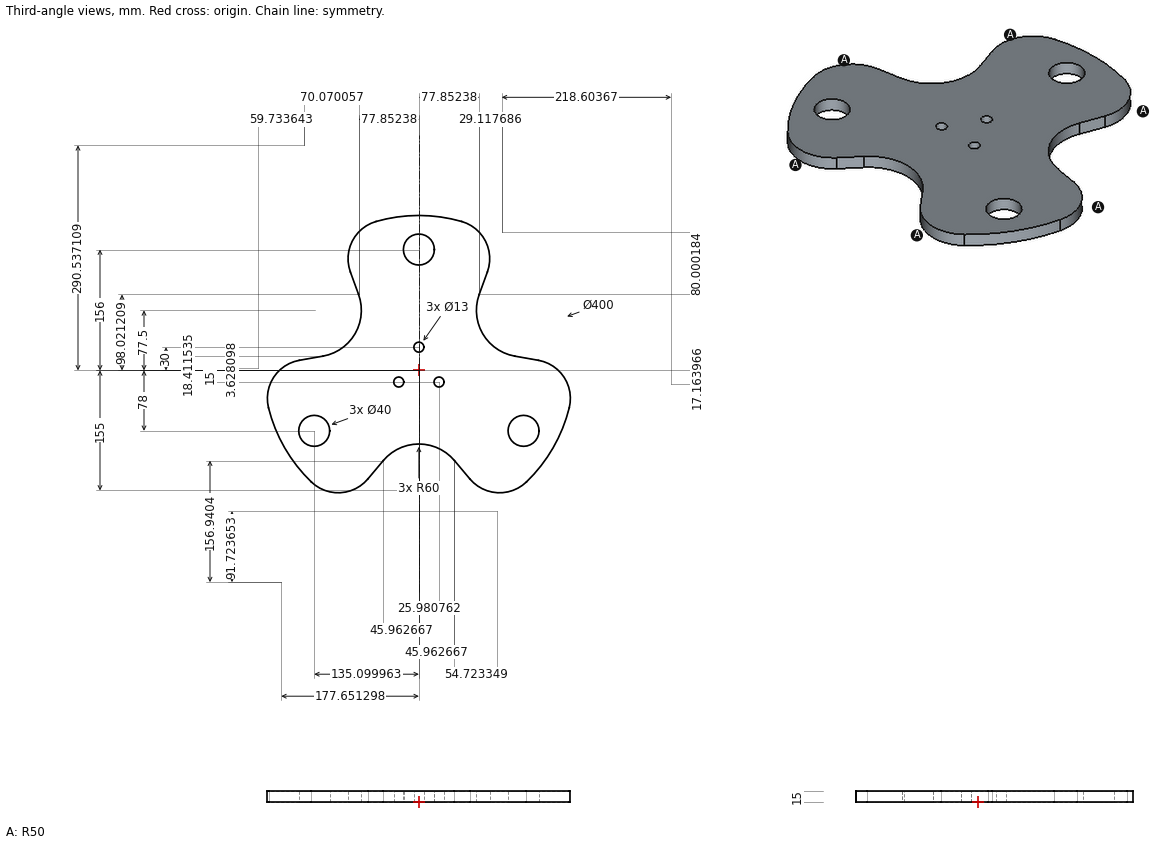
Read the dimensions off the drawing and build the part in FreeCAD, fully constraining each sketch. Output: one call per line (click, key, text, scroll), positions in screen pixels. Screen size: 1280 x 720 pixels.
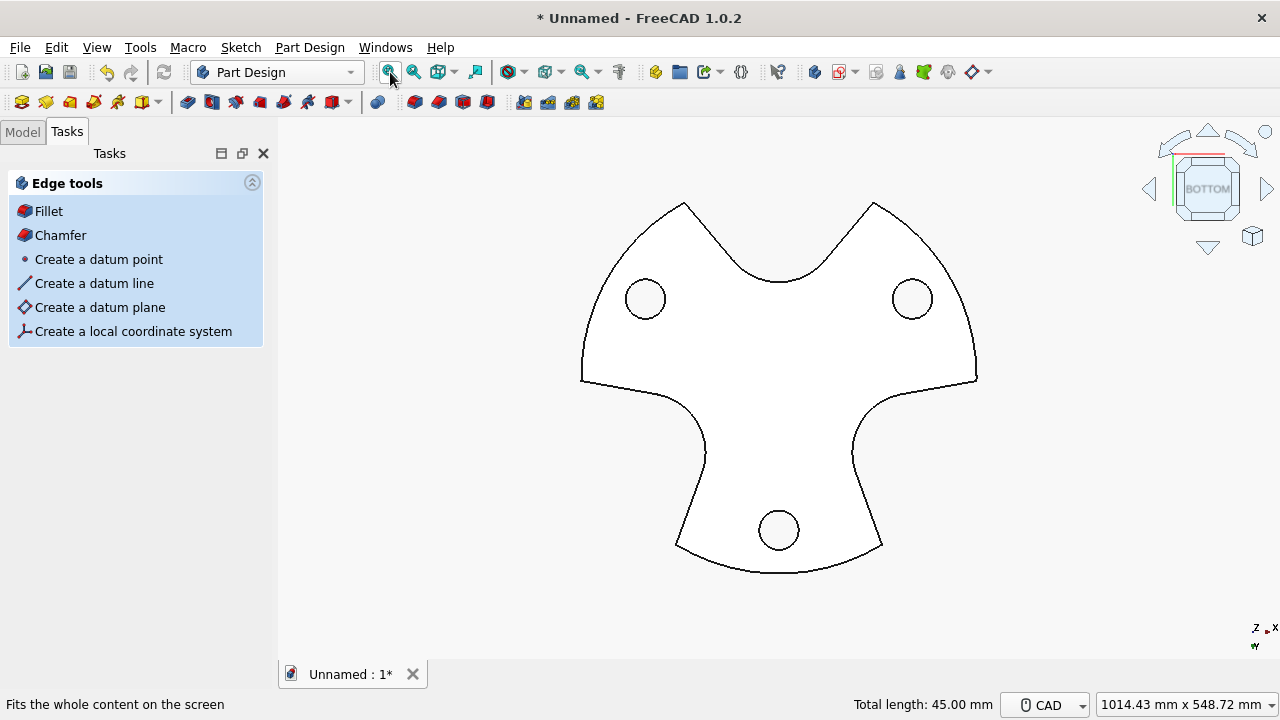
key(4)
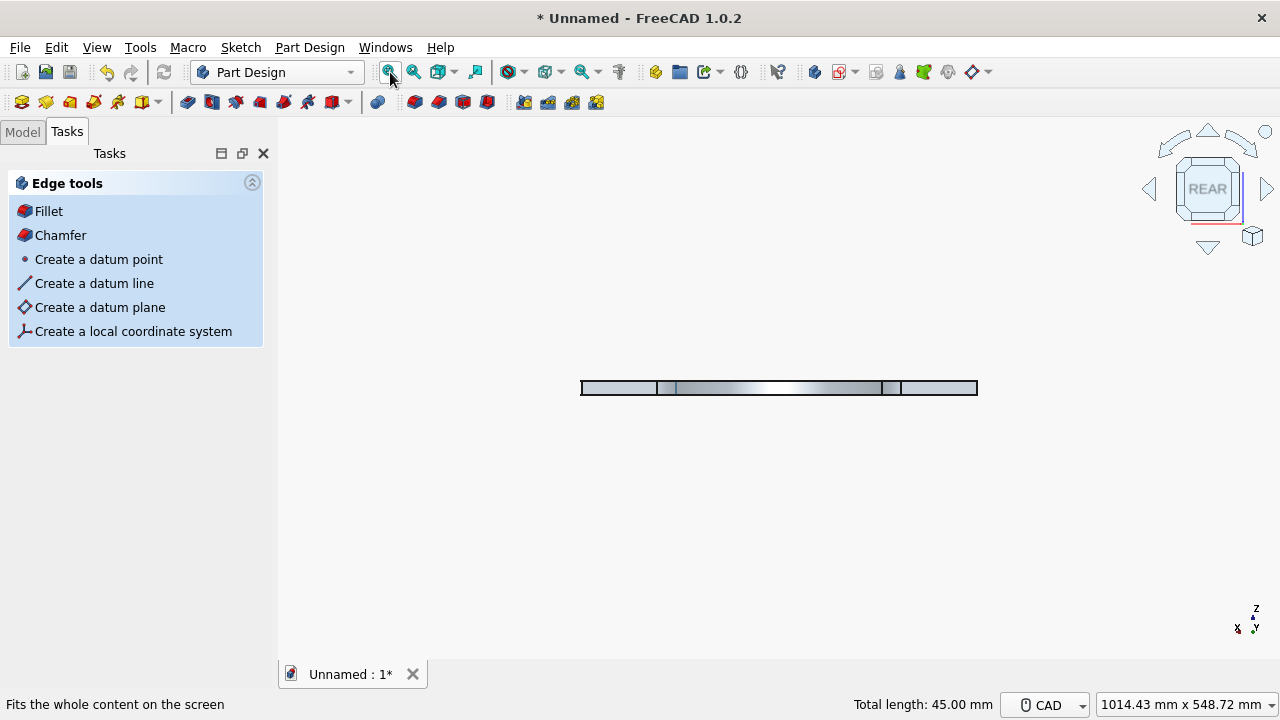
click(390, 72)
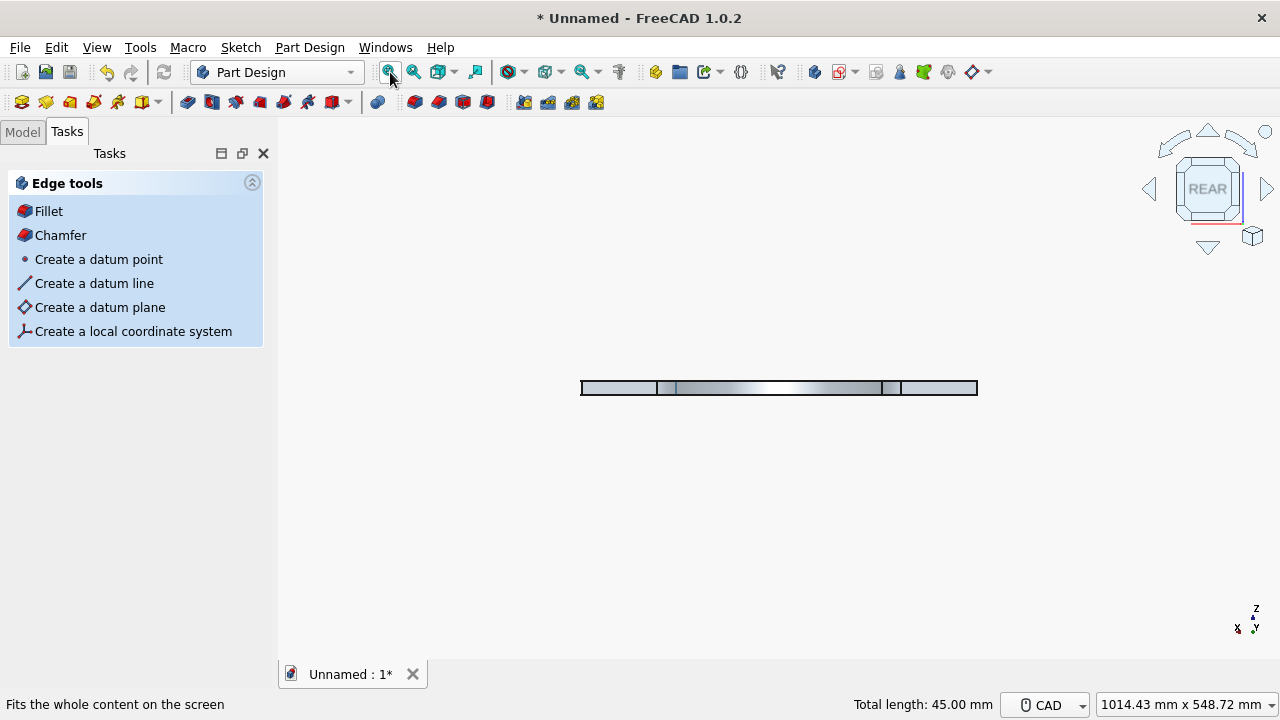
scroll(582, 387, up, 5)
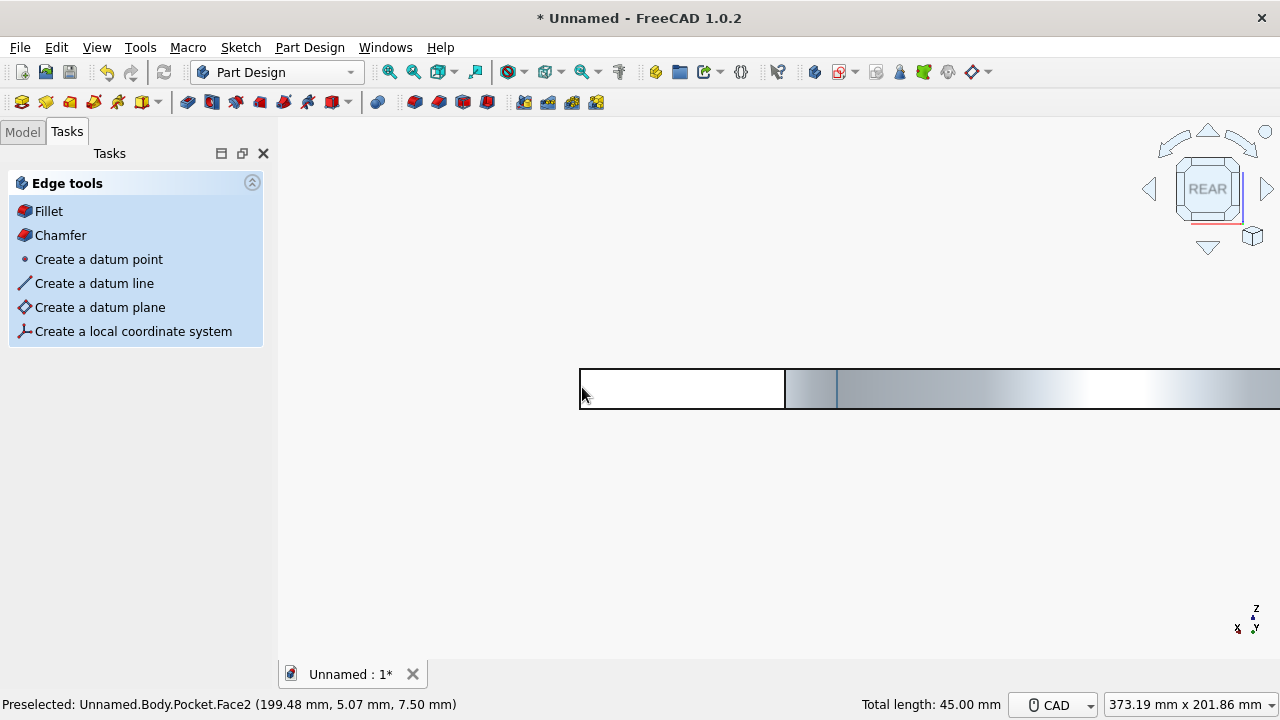
click(390, 72)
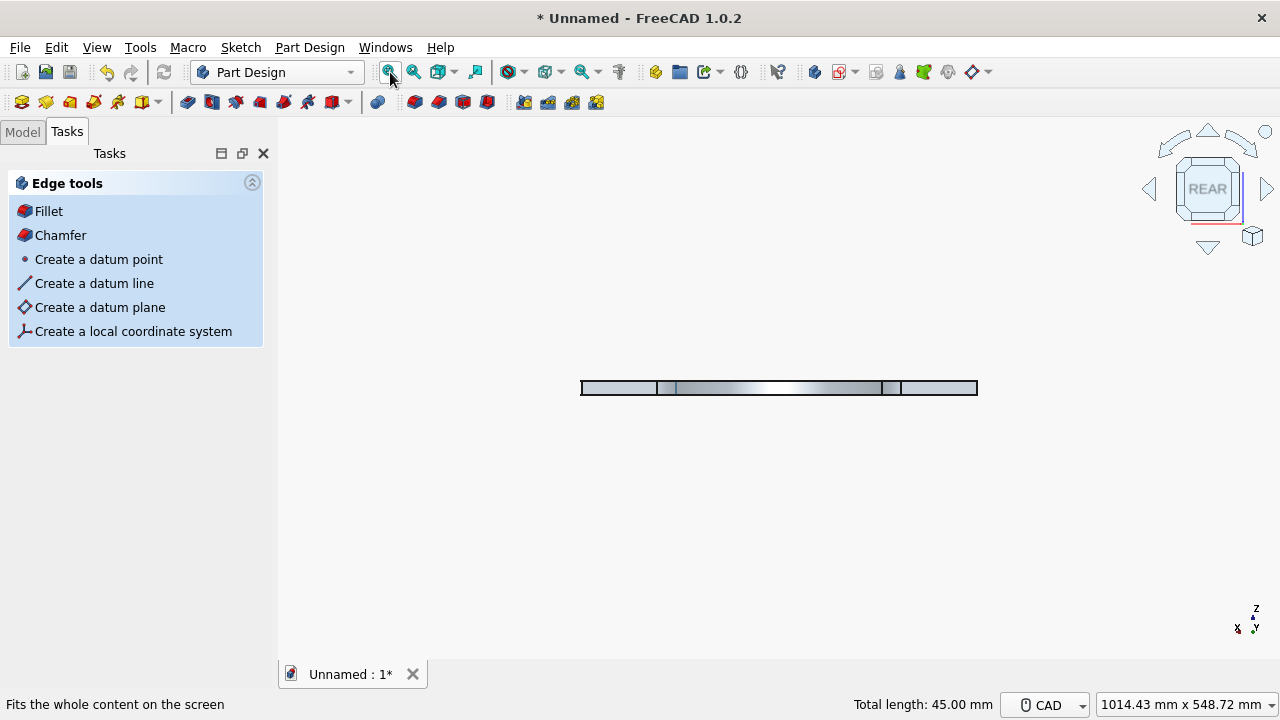
key(6)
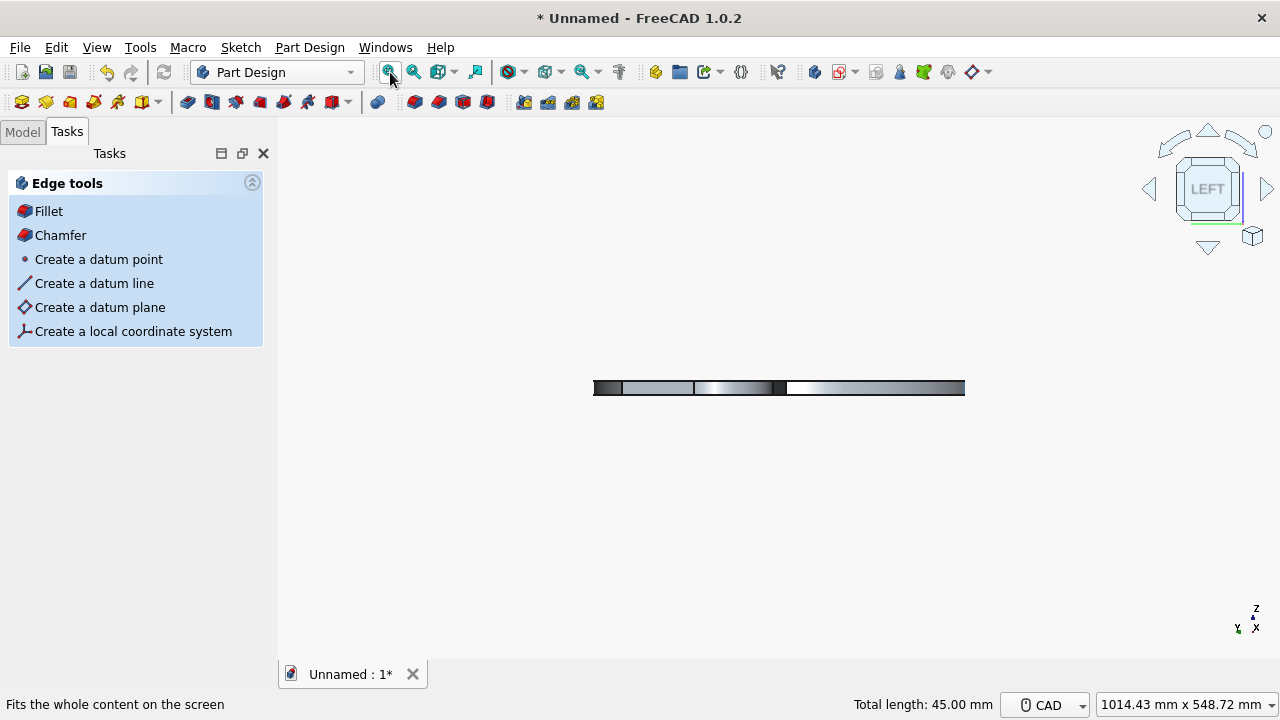
click(390, 72)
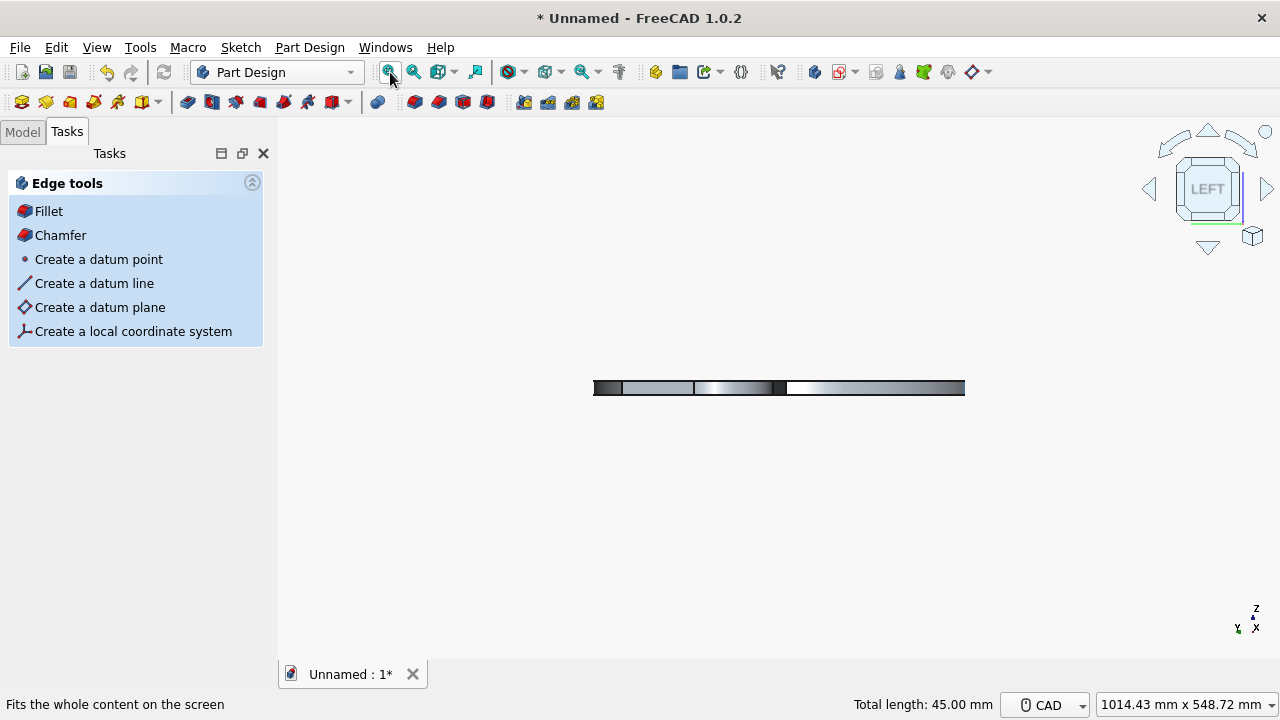
click(622, 387, ctrl)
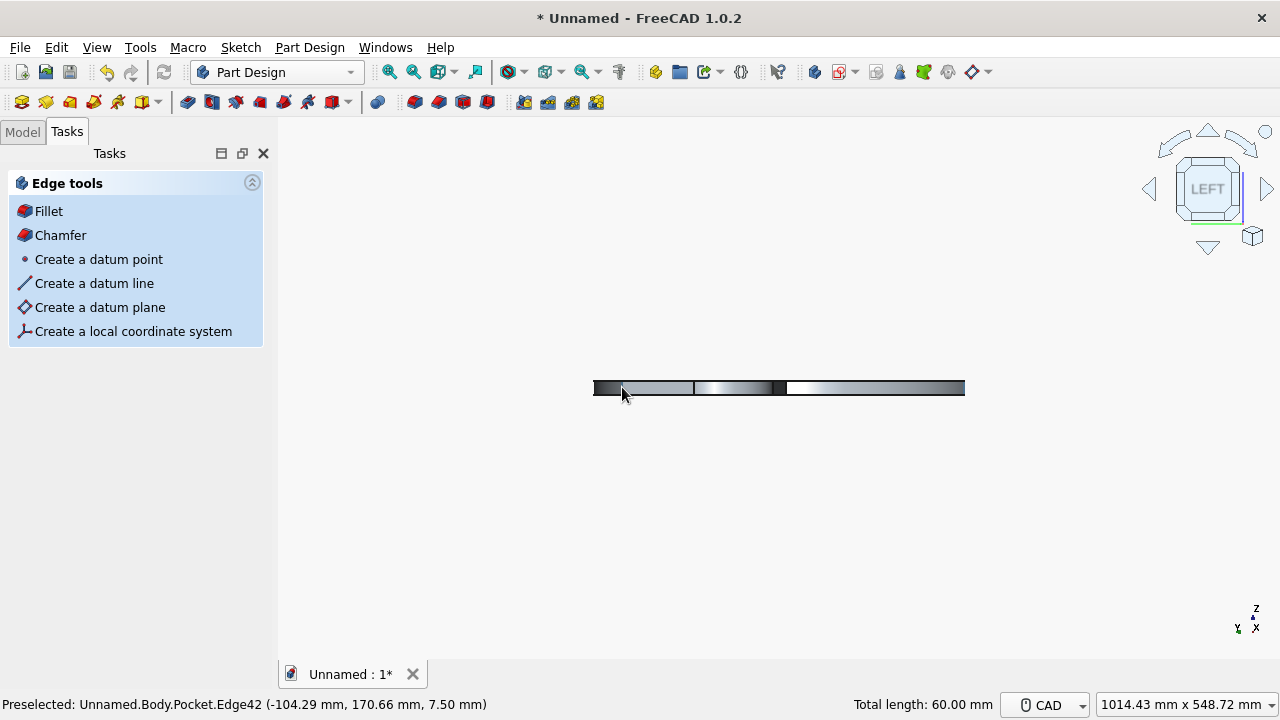
click(786, 387, ctrl)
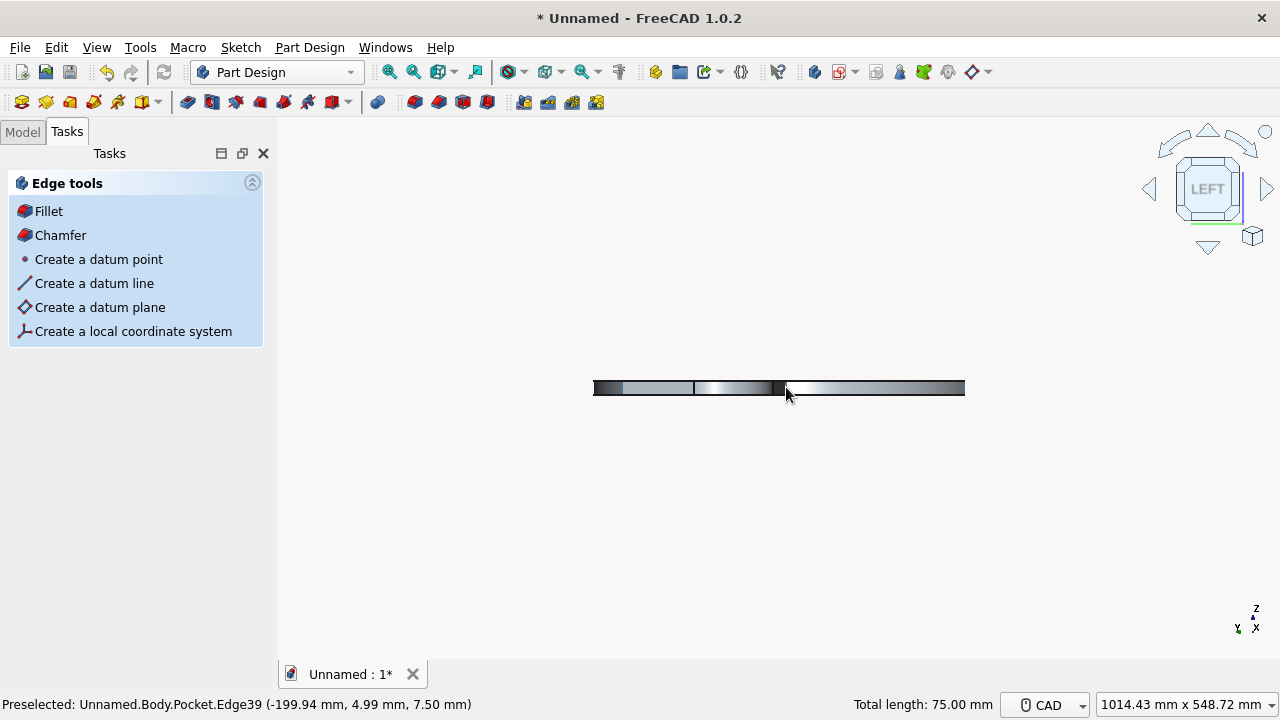
scroll(786, 387, up, 5)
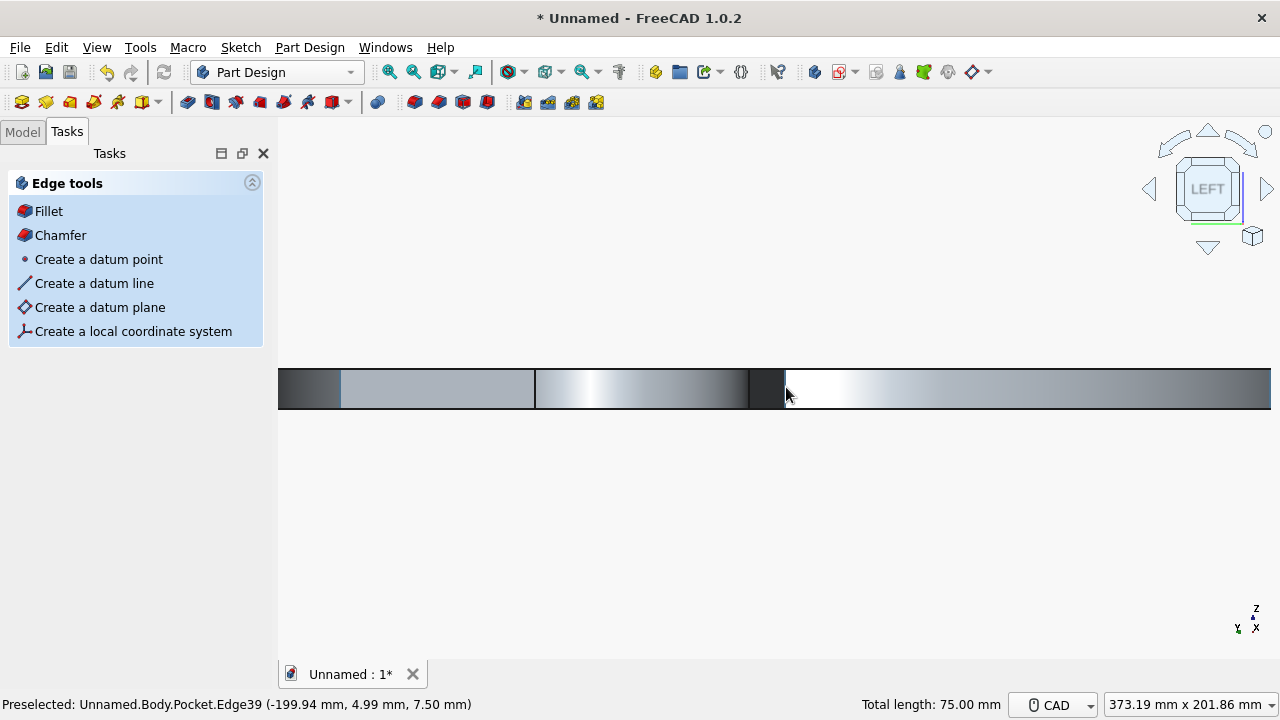
click(390, 72)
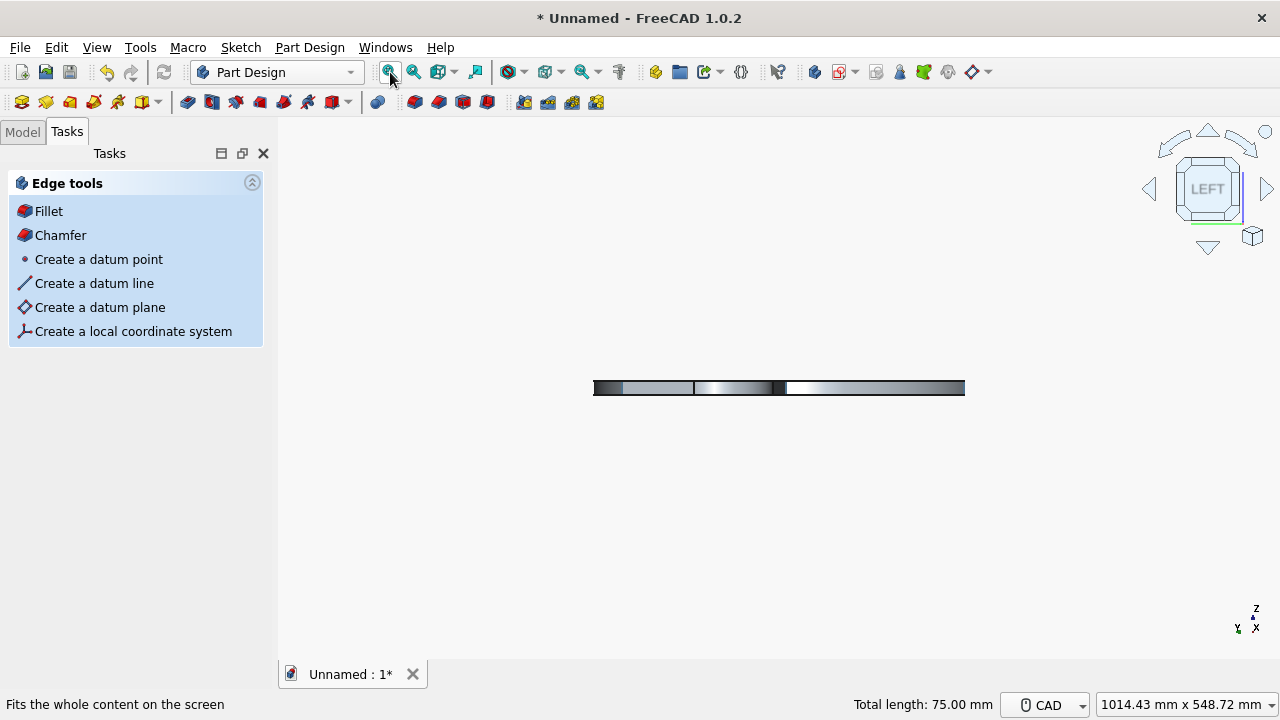
key(v)
key(3)